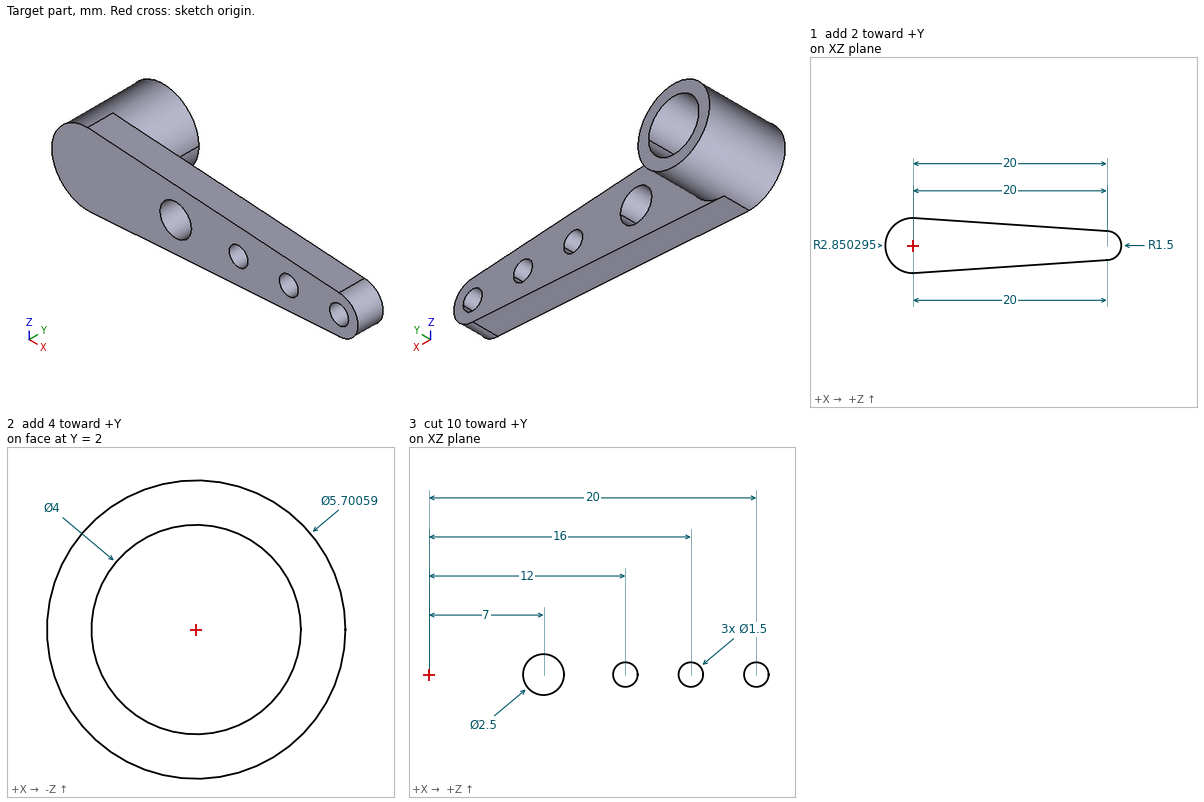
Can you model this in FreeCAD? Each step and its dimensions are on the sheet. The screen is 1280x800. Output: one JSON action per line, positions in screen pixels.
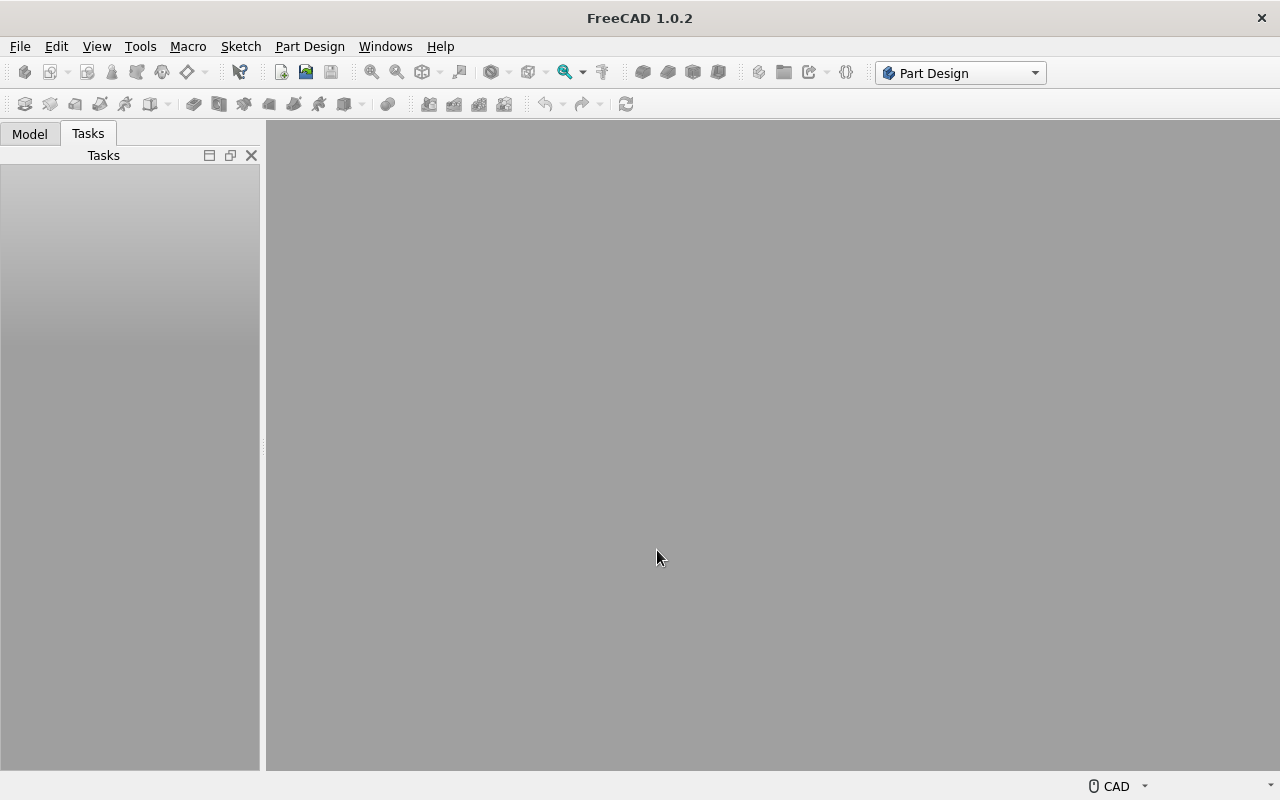
{"action": "left_click", "coordinate": [281, 72]}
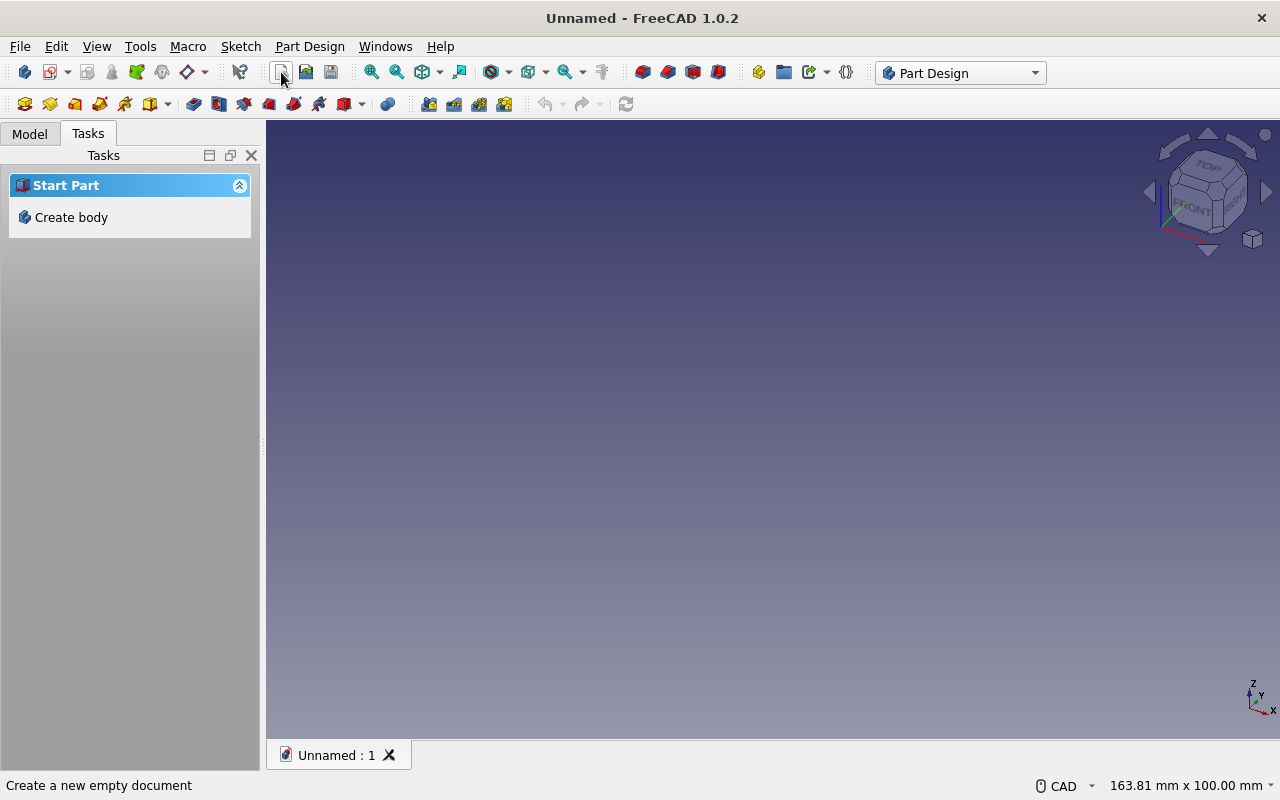
{"action": "left_click", "coordinate": [50, 72]}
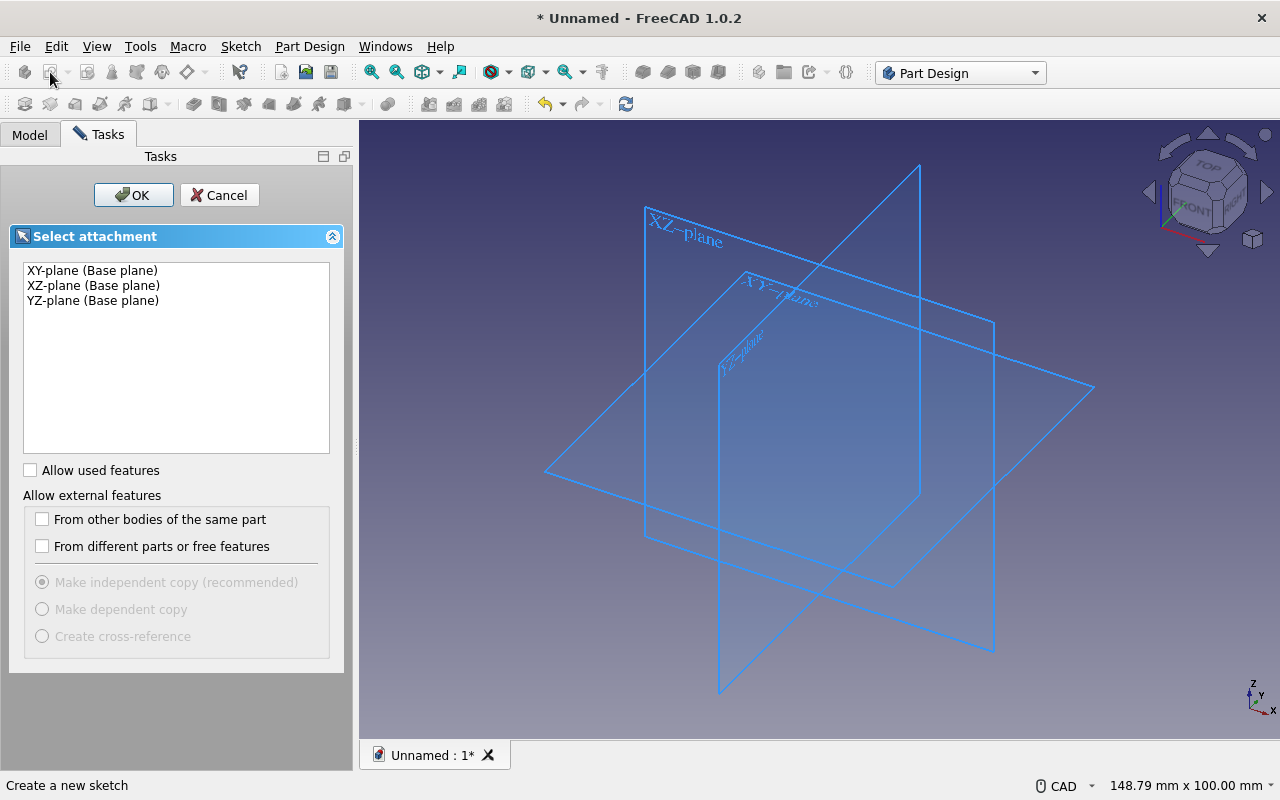
{"action": "left_click", "coordinate": [84, 286]}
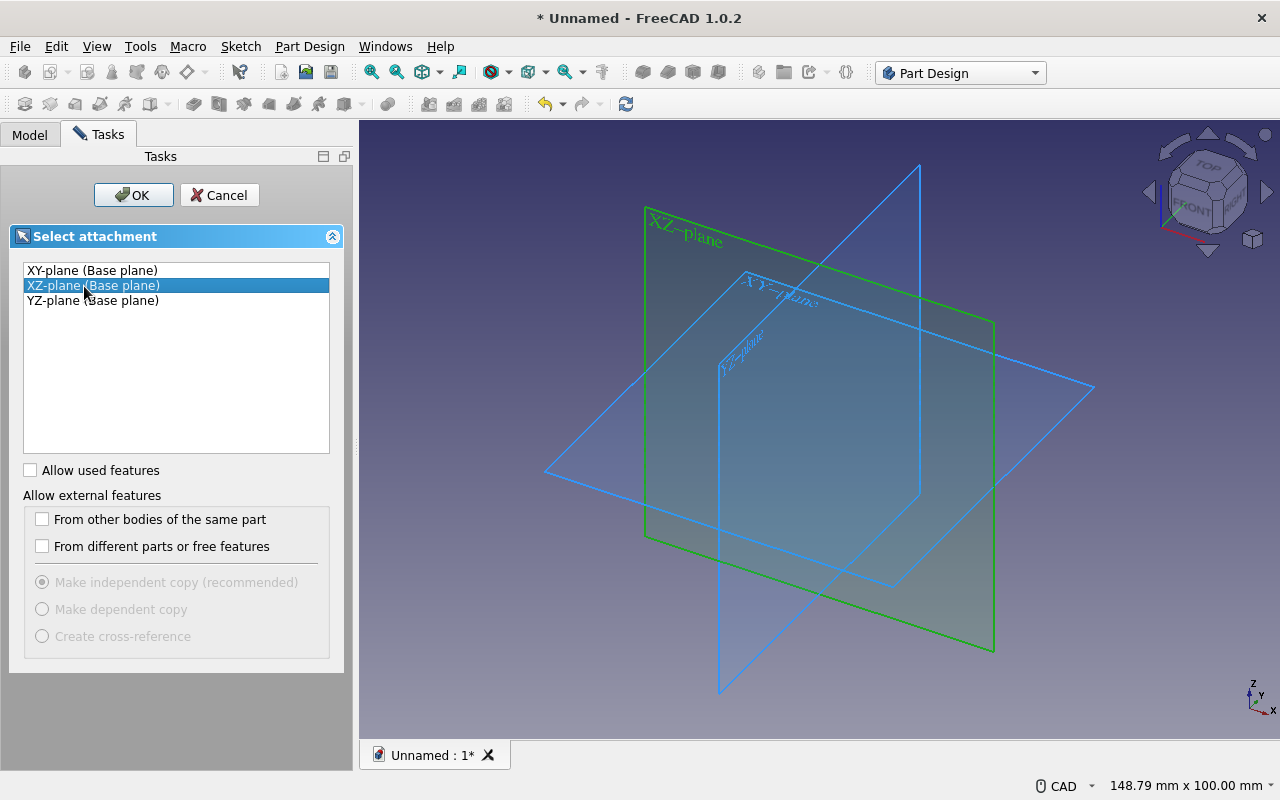
{"action": "left_click", "coordinate": [134, 195]}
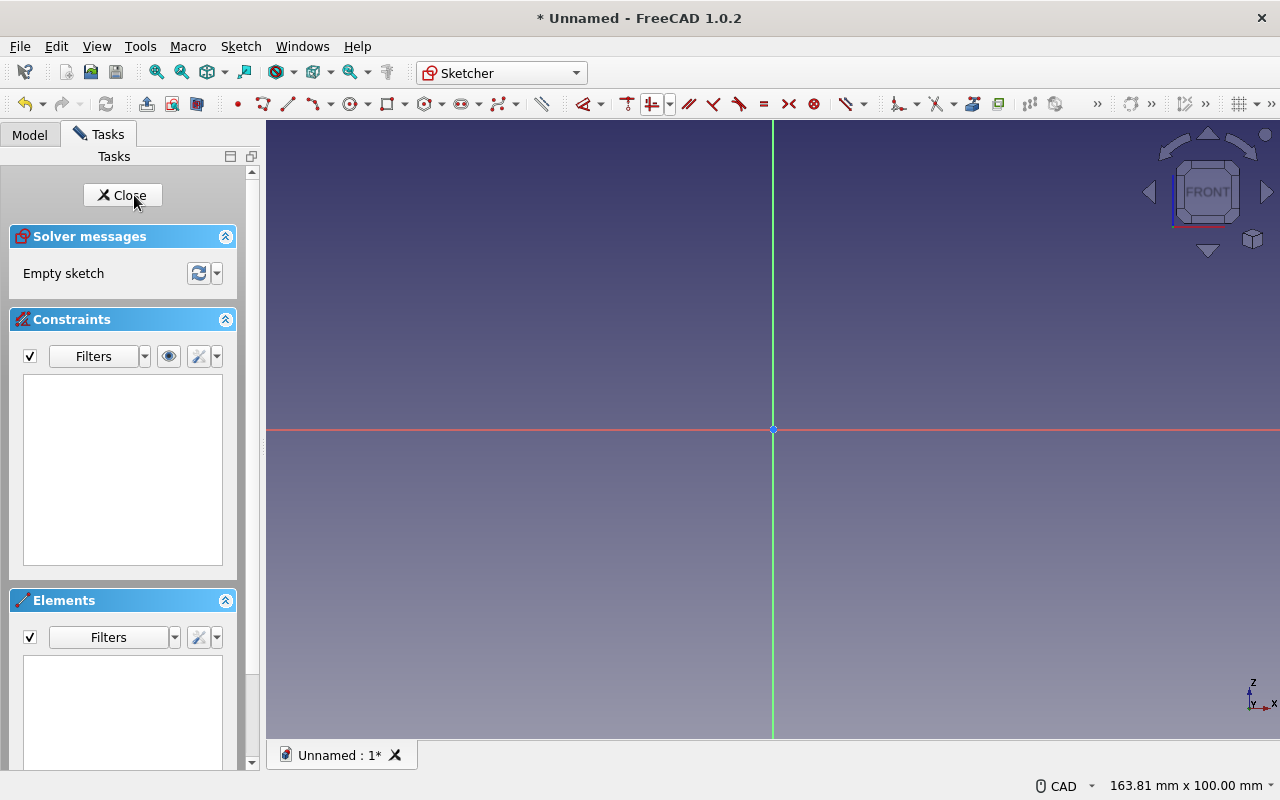
{"action": "scroll", "coordinate": [872, 430], "scroll_direction": "up", "scroll_amount": 7}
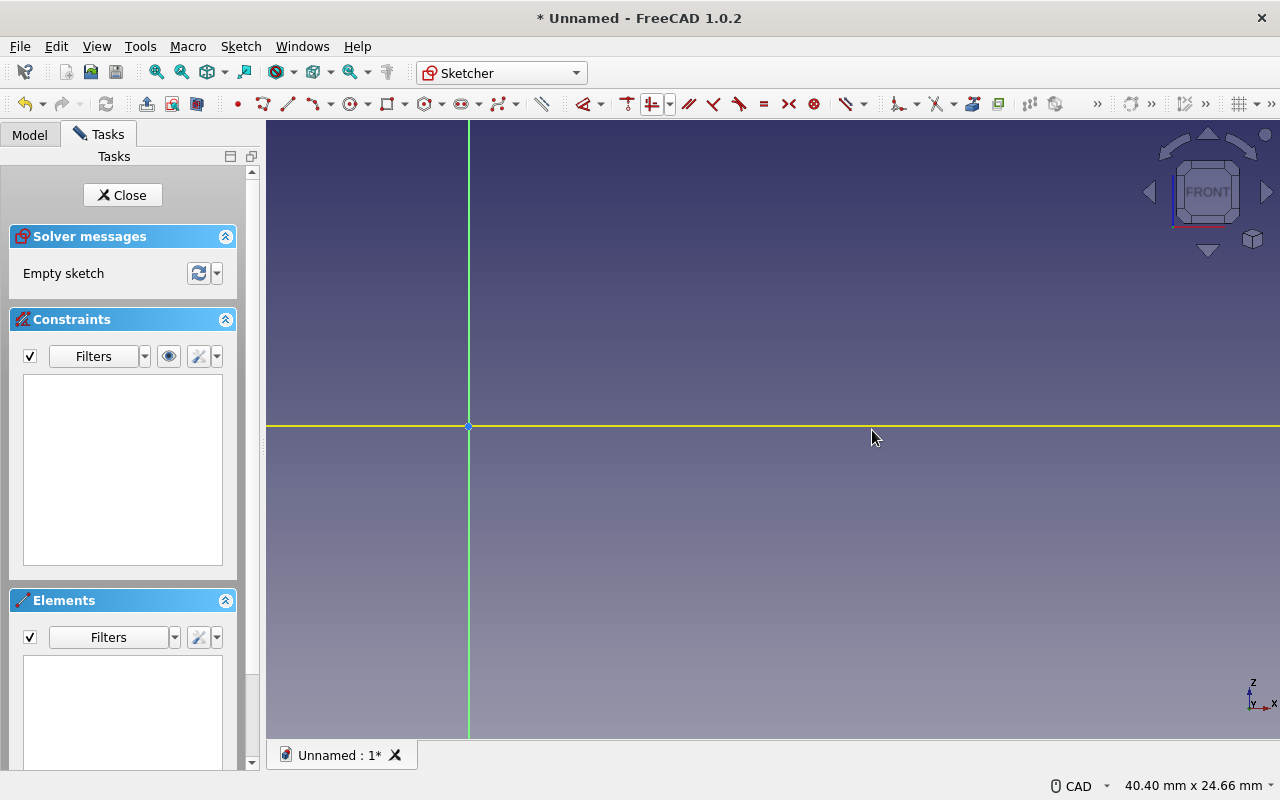
{"action": "left_click", "coordinate": [288, 104]}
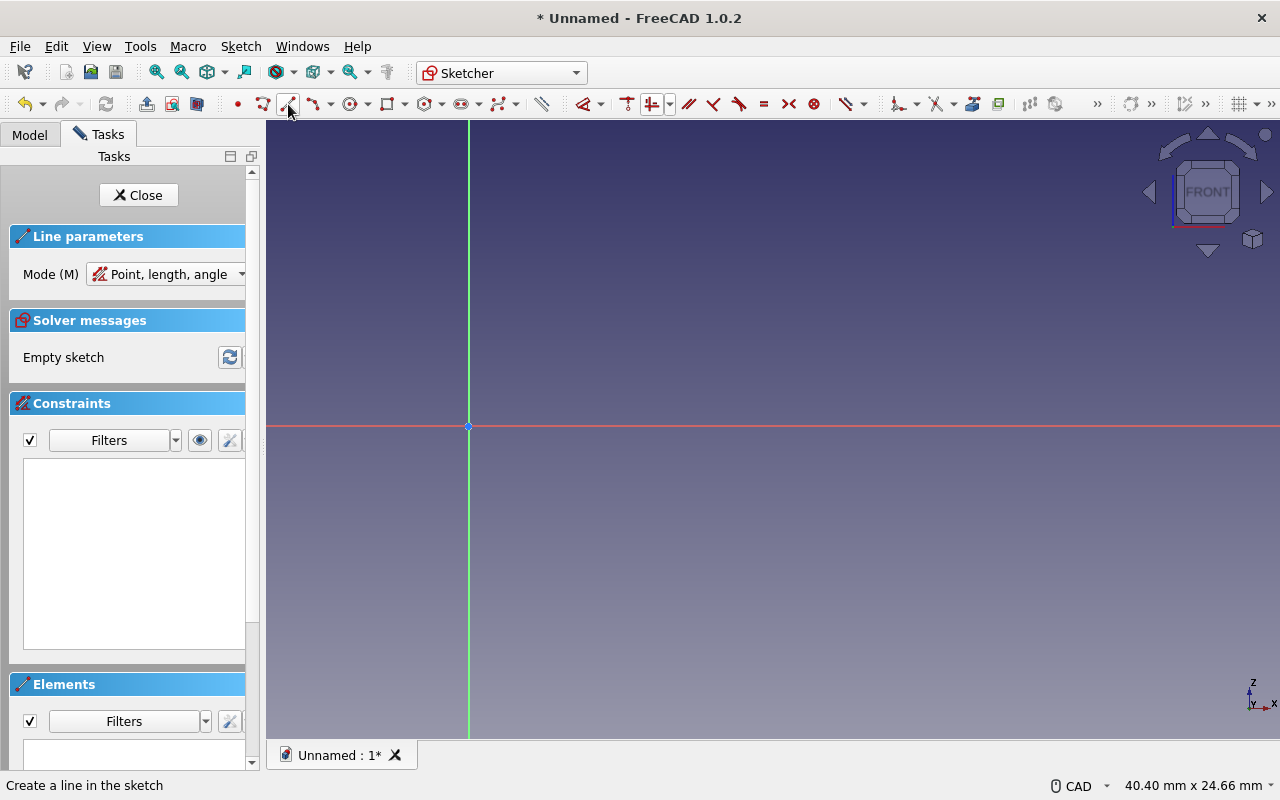
{"action": "left_click", "coordinate": [971, 464]}
{"action": "left_click", "coordinate": [469, 498]}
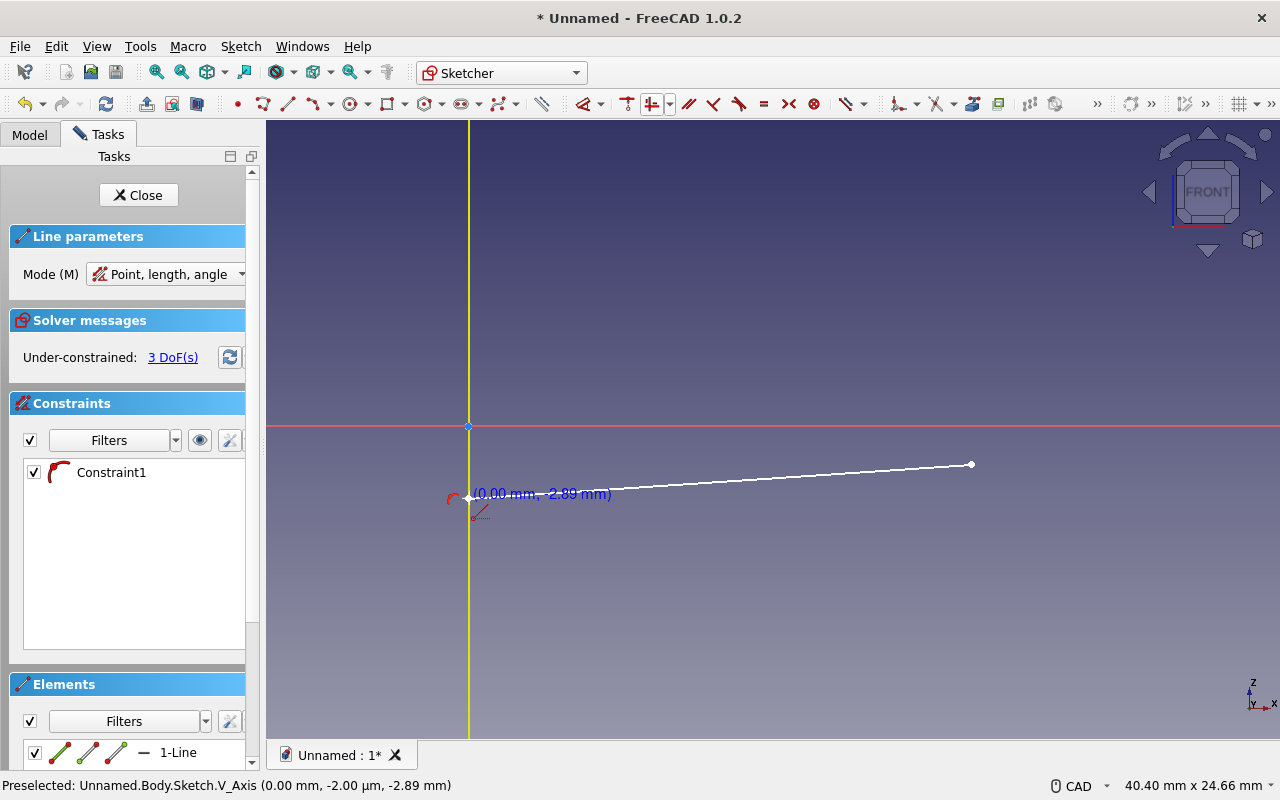
{"action": "left_click", "coordinate": [469, 355]}
{"action": "left_click", "coordinate": [971, 389]}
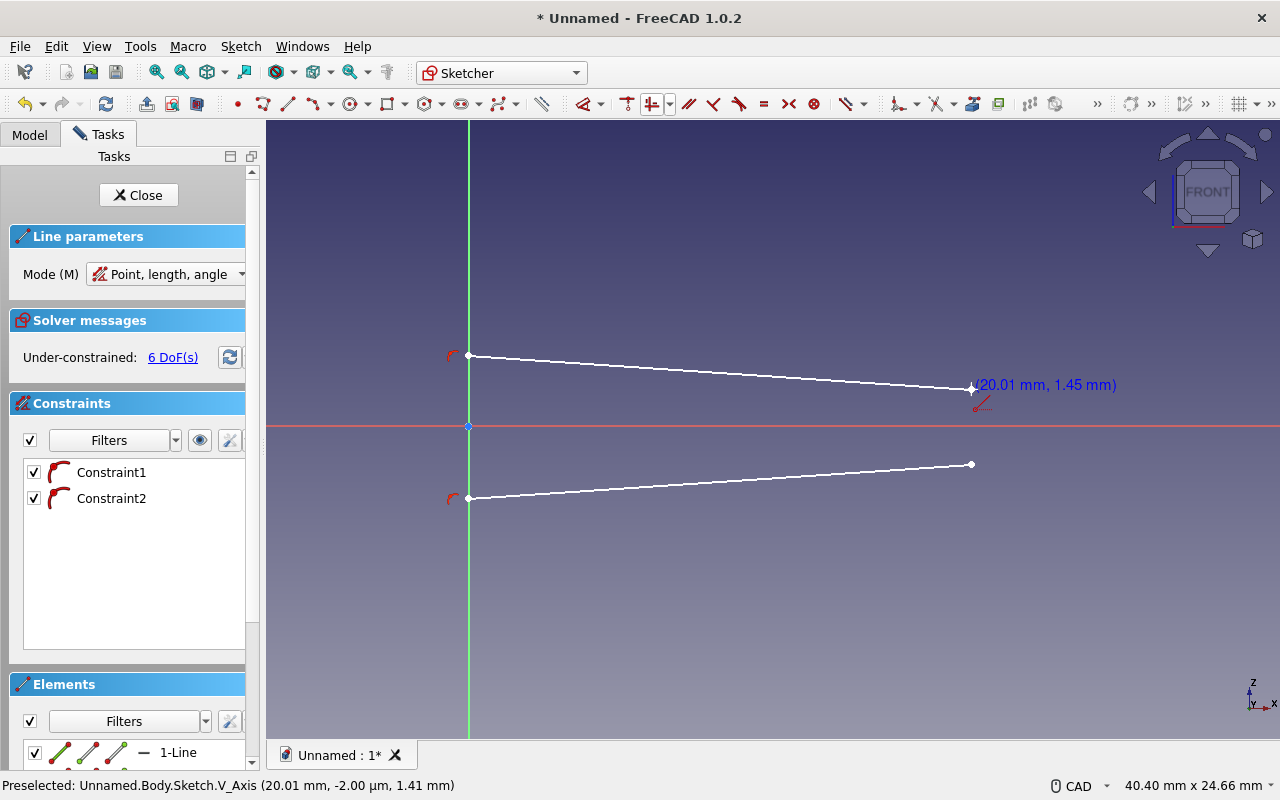
{"action": "left_click", "coordinate": [312, 104]}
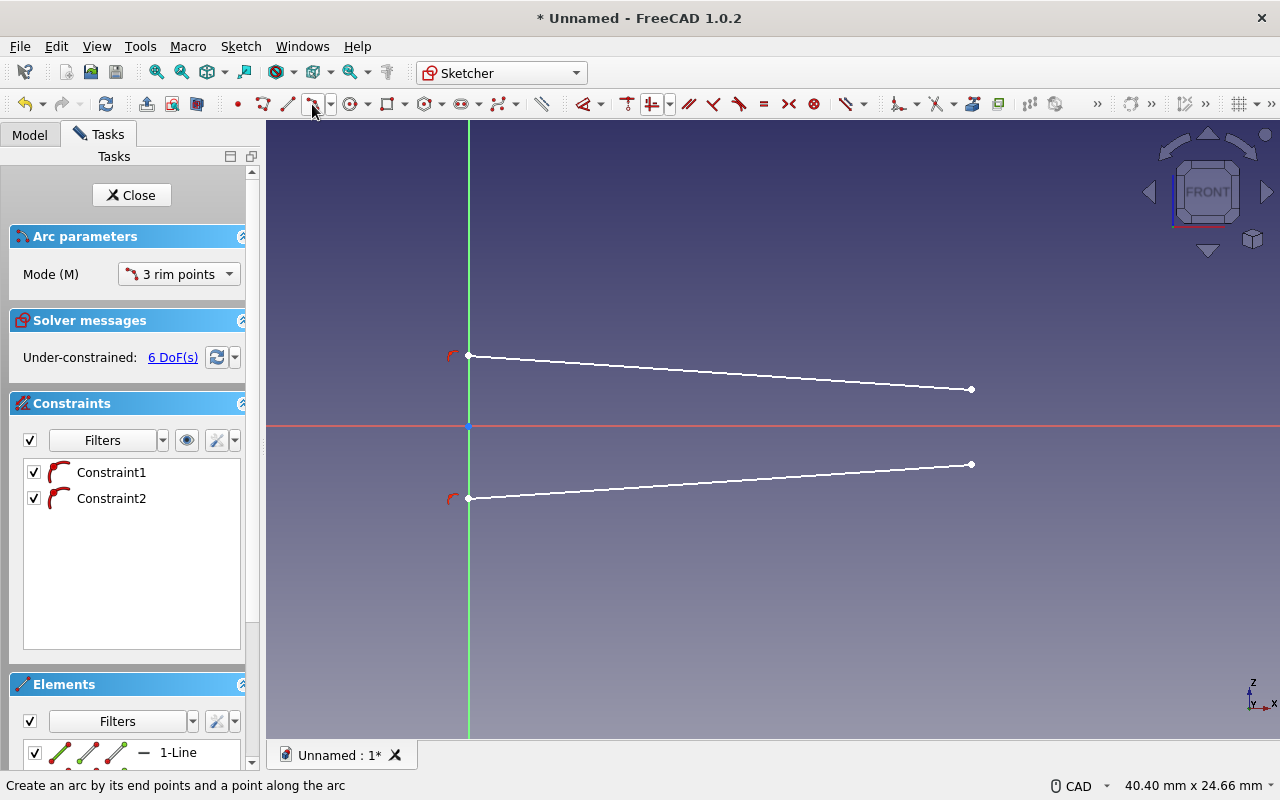
{"action": "left_click", "coordinate": [469, 499]}
{"action": "left_click", "coordinate": [469, 356]}
{"action": "left_click", "coordinate": [401, 404]}